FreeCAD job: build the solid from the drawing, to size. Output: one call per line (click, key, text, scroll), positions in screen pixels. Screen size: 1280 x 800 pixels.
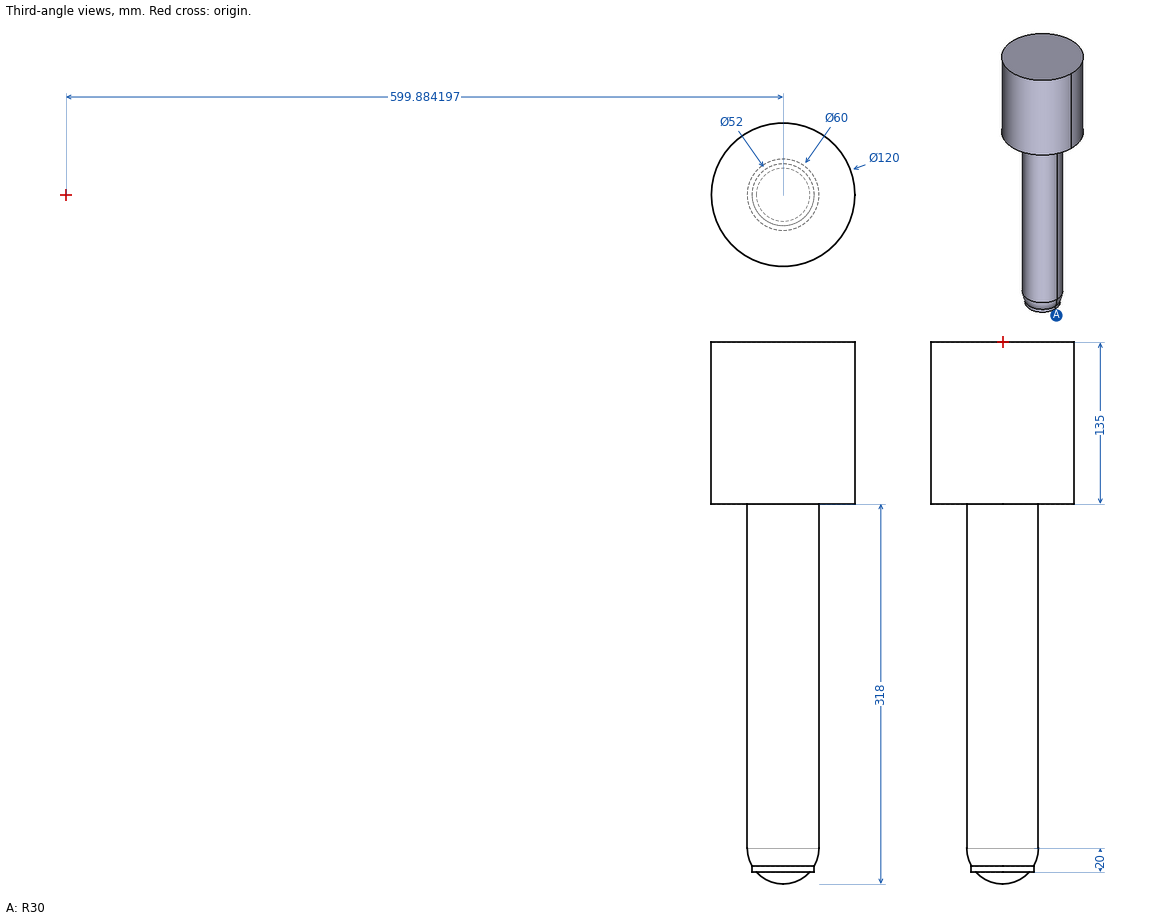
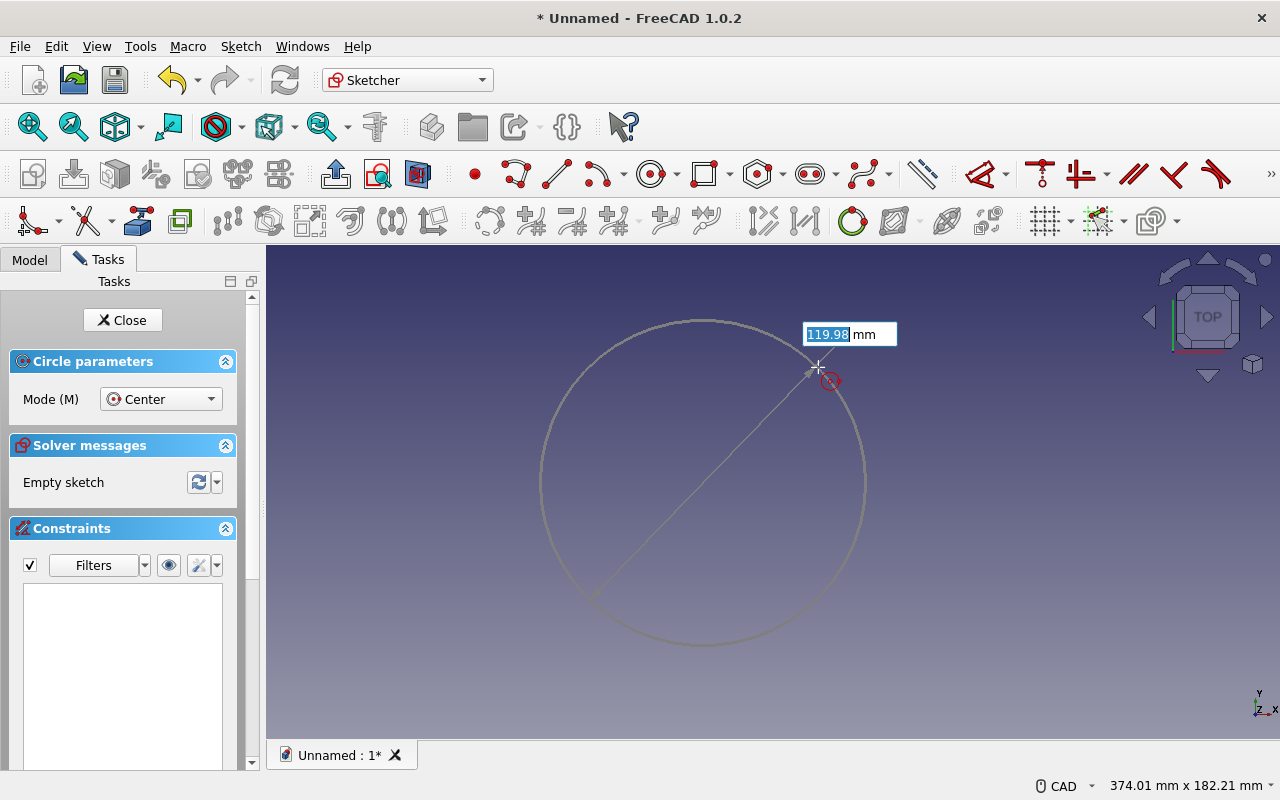
text(120)
key(Return)
key(Escape)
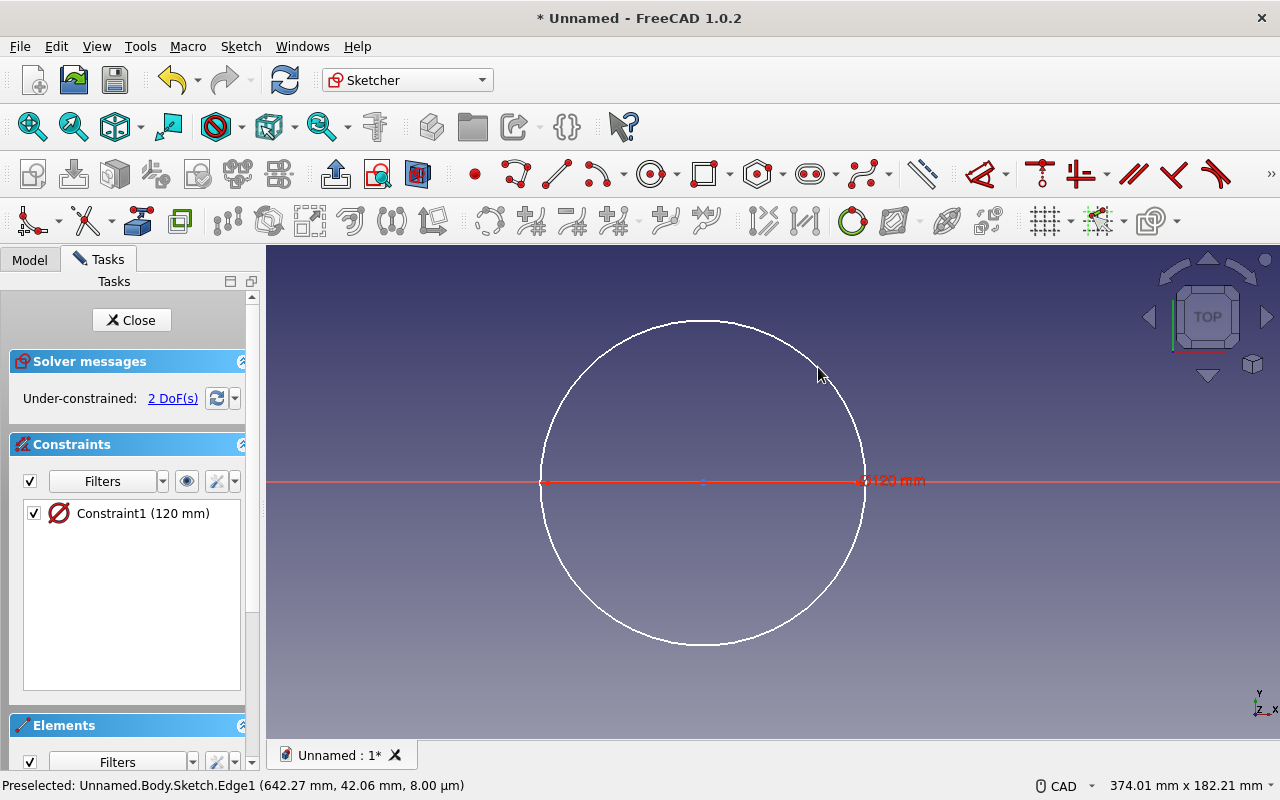
click(703, 483)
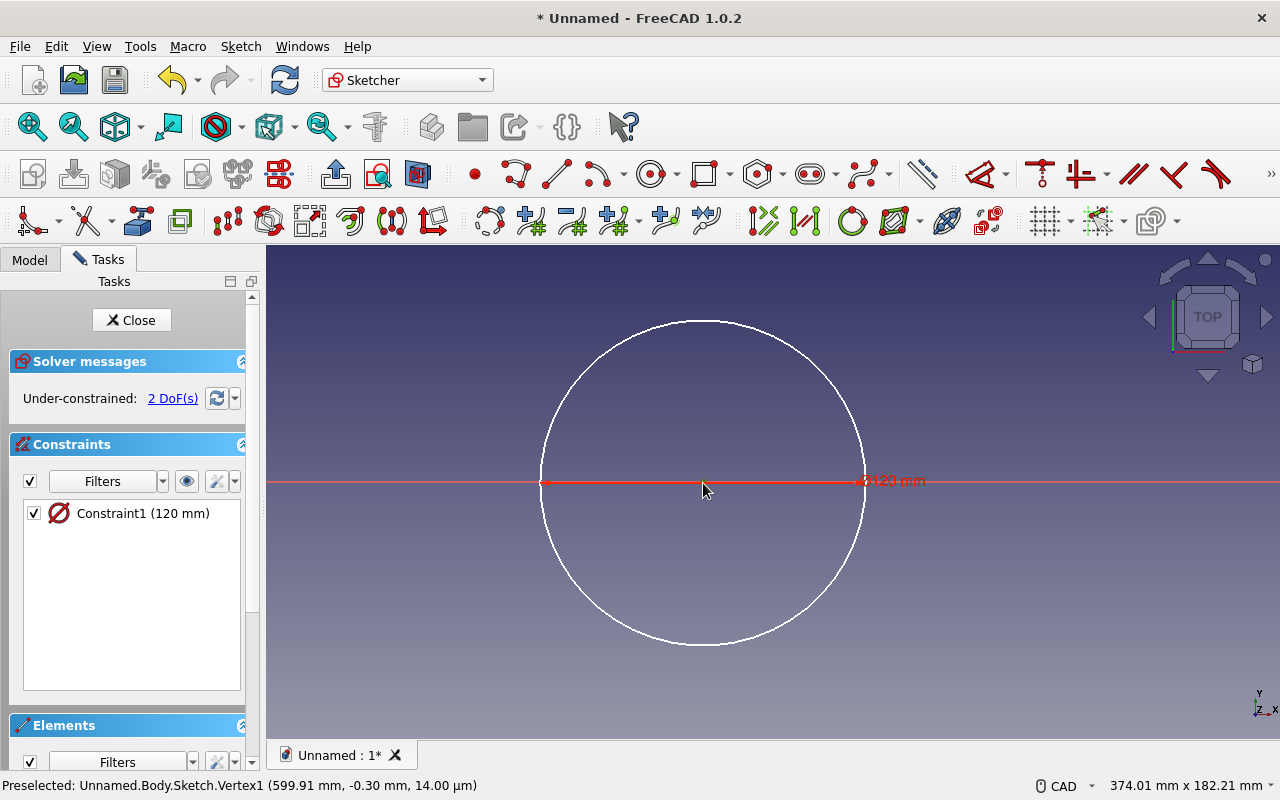
click(353, 482)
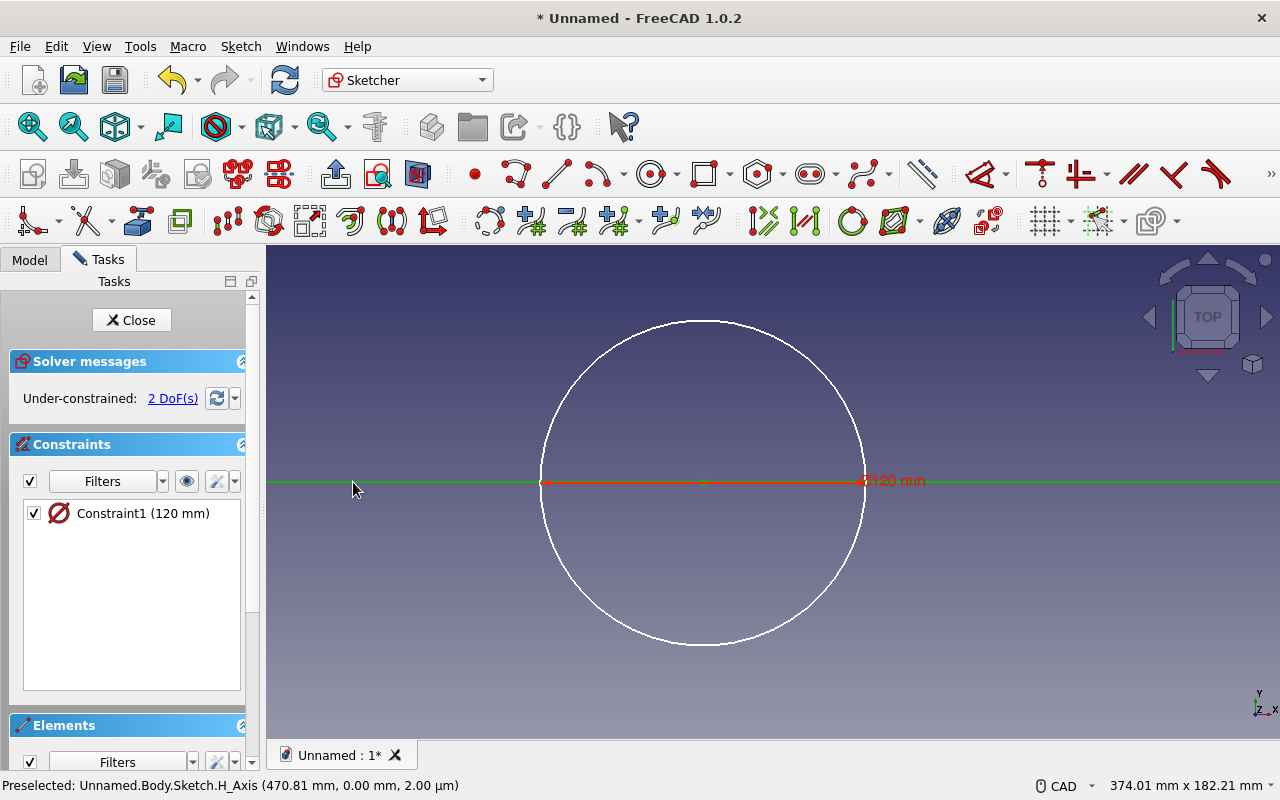
click(1040, 174)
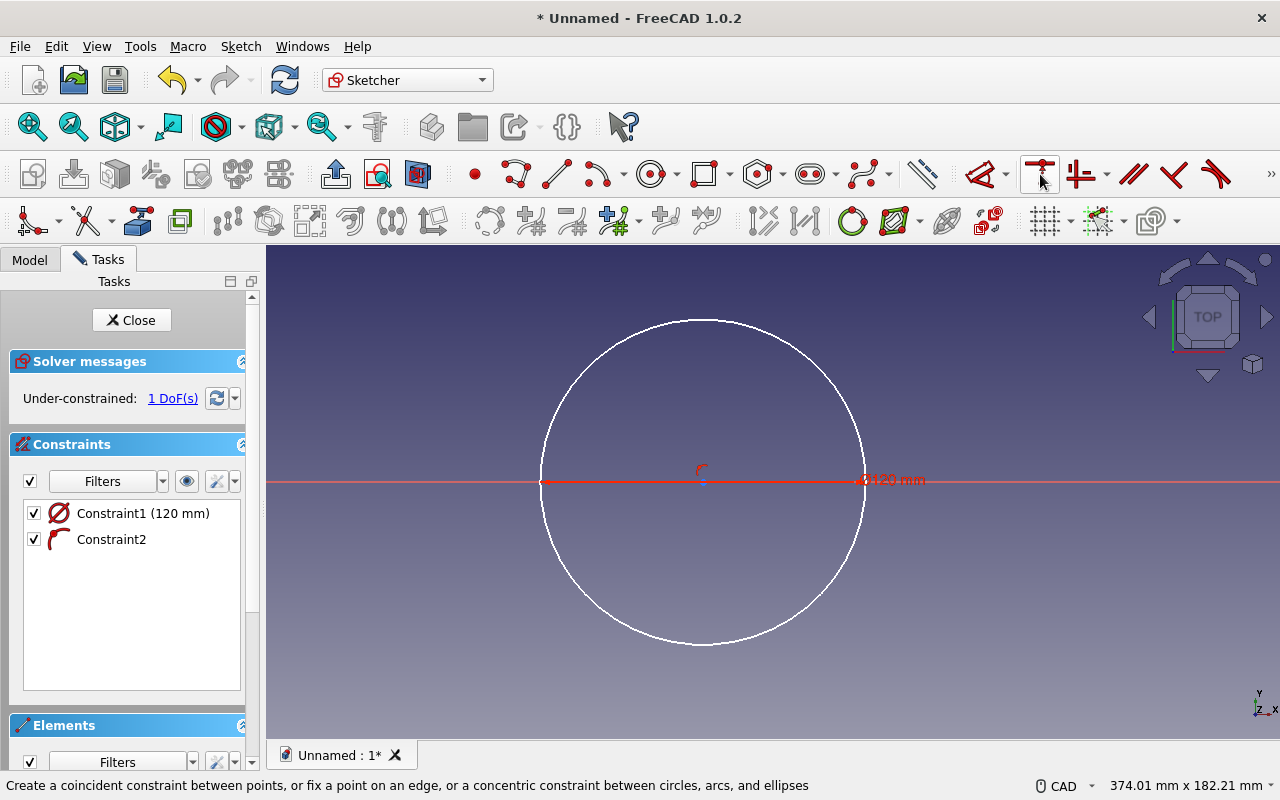
click(980, 174)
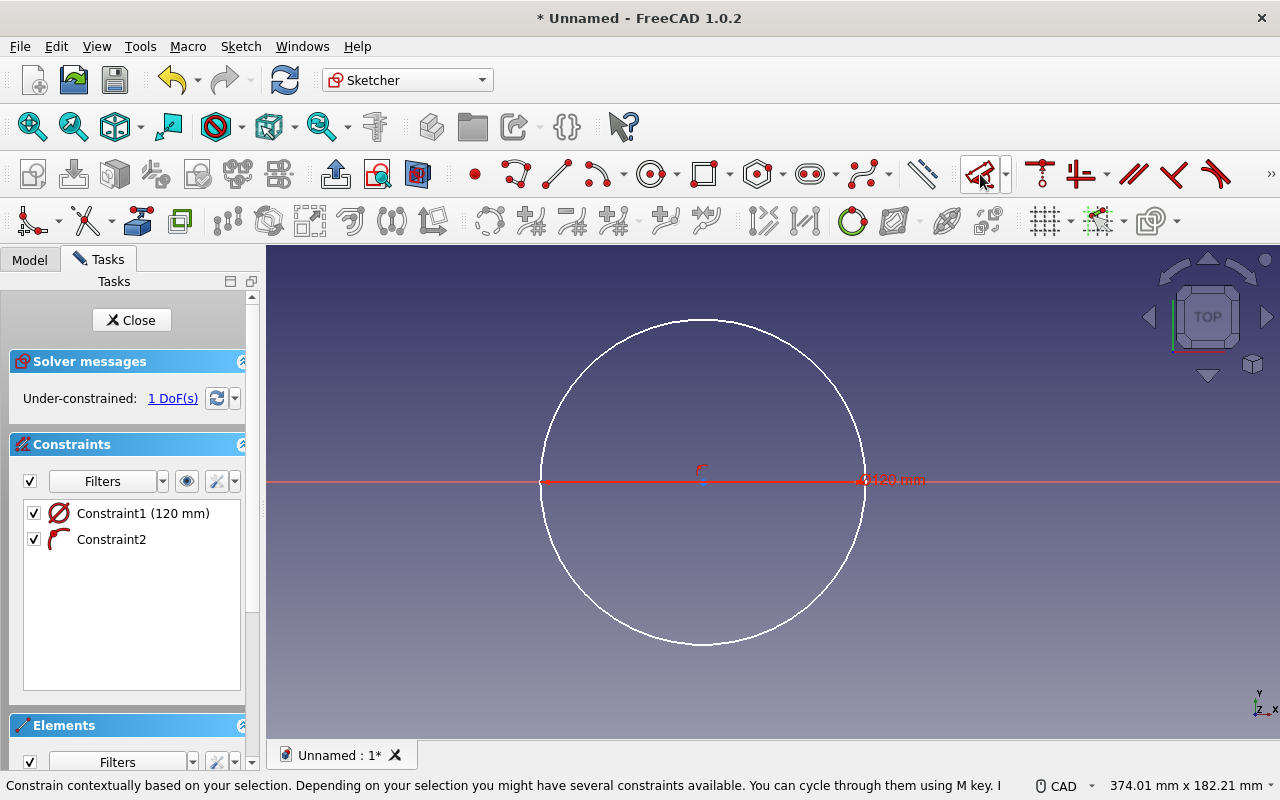
click(703, 482)
click(498, 516)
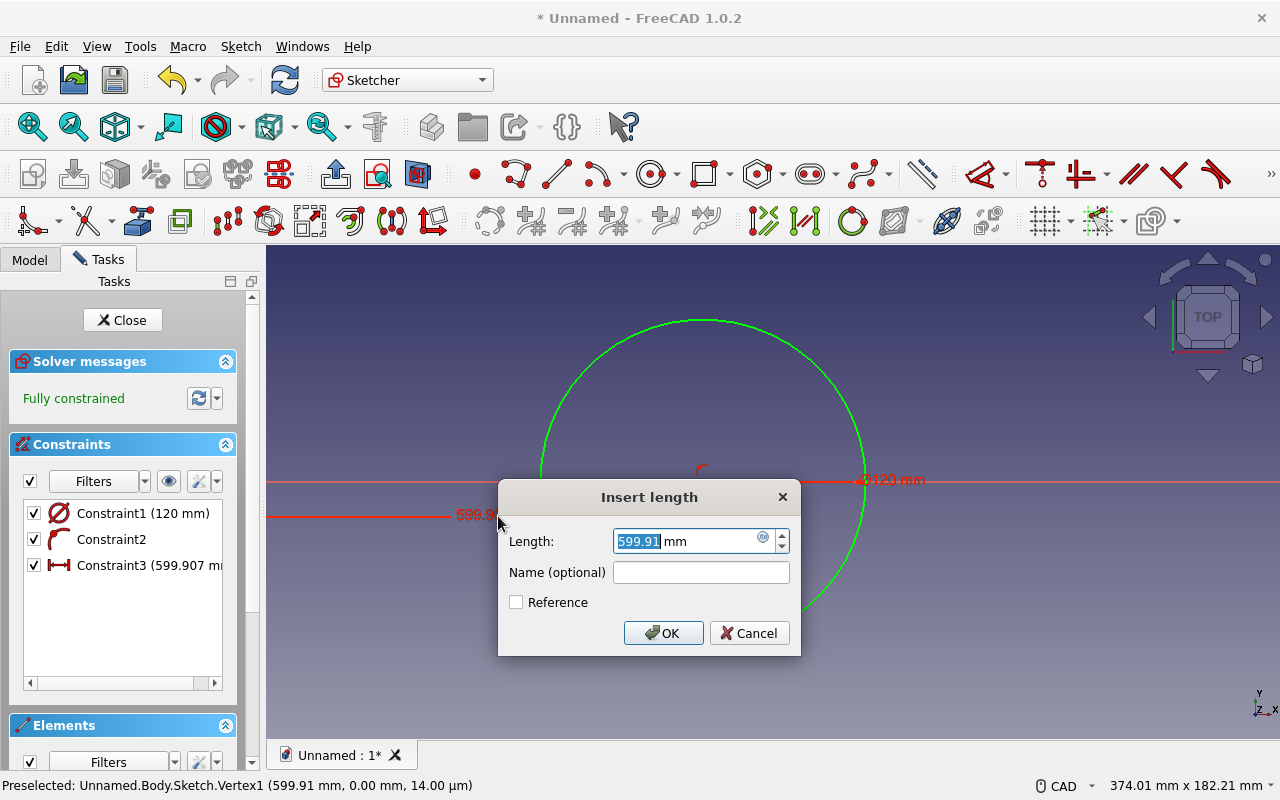
text(599.884197)
key(Return)
key(Escape)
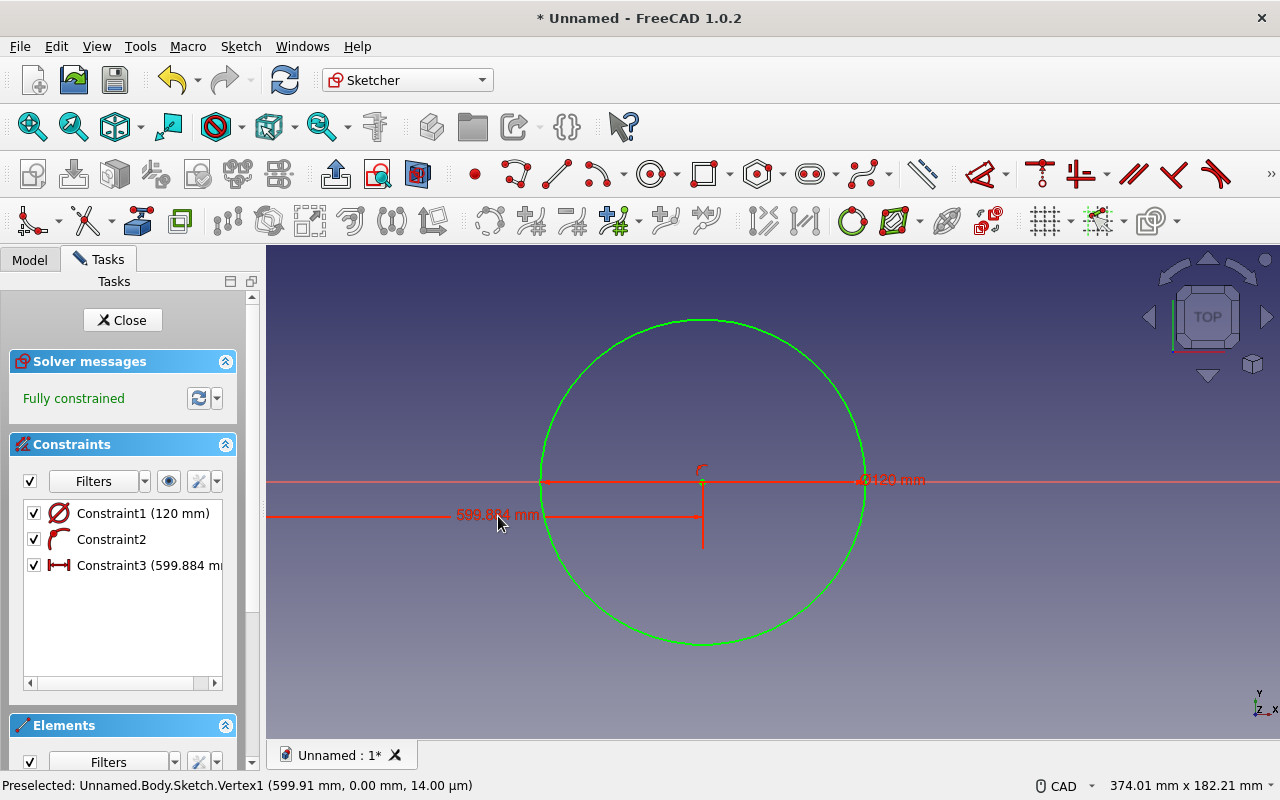
click(123, 320)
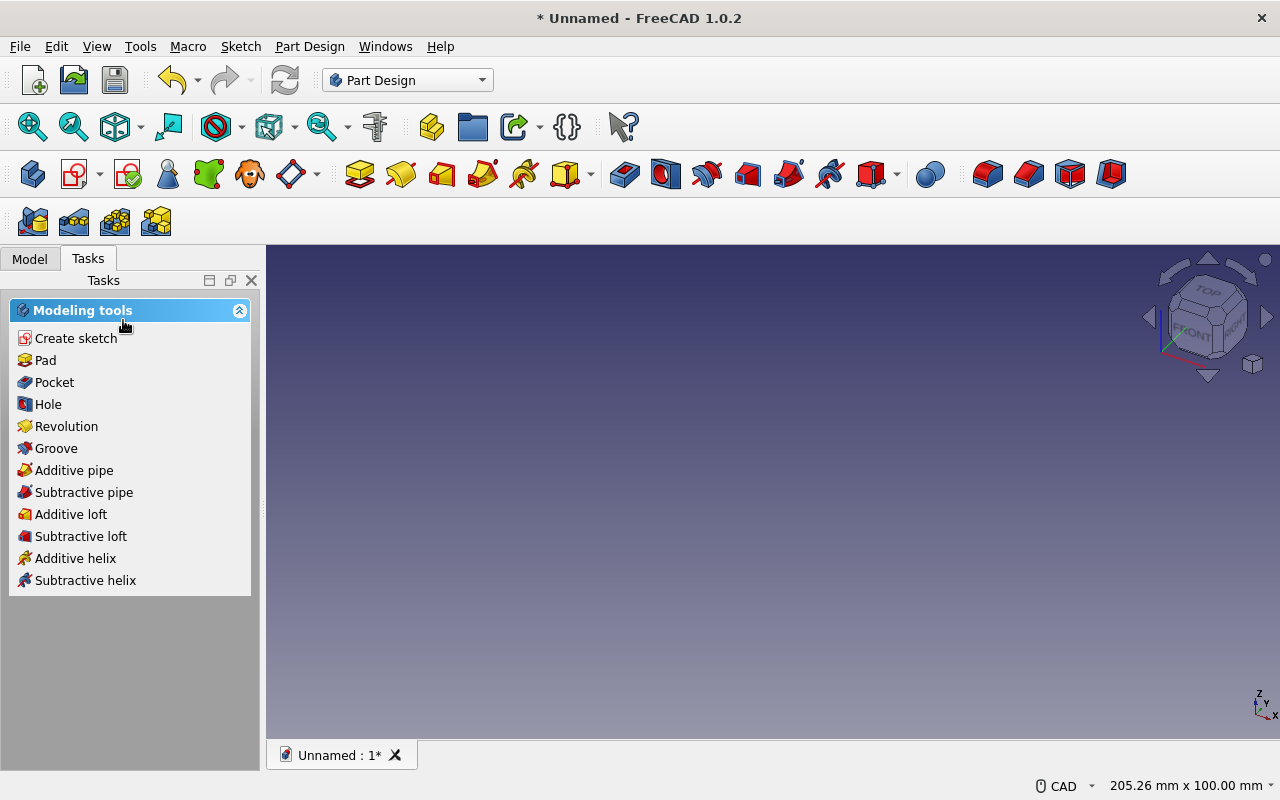
click(360, 174)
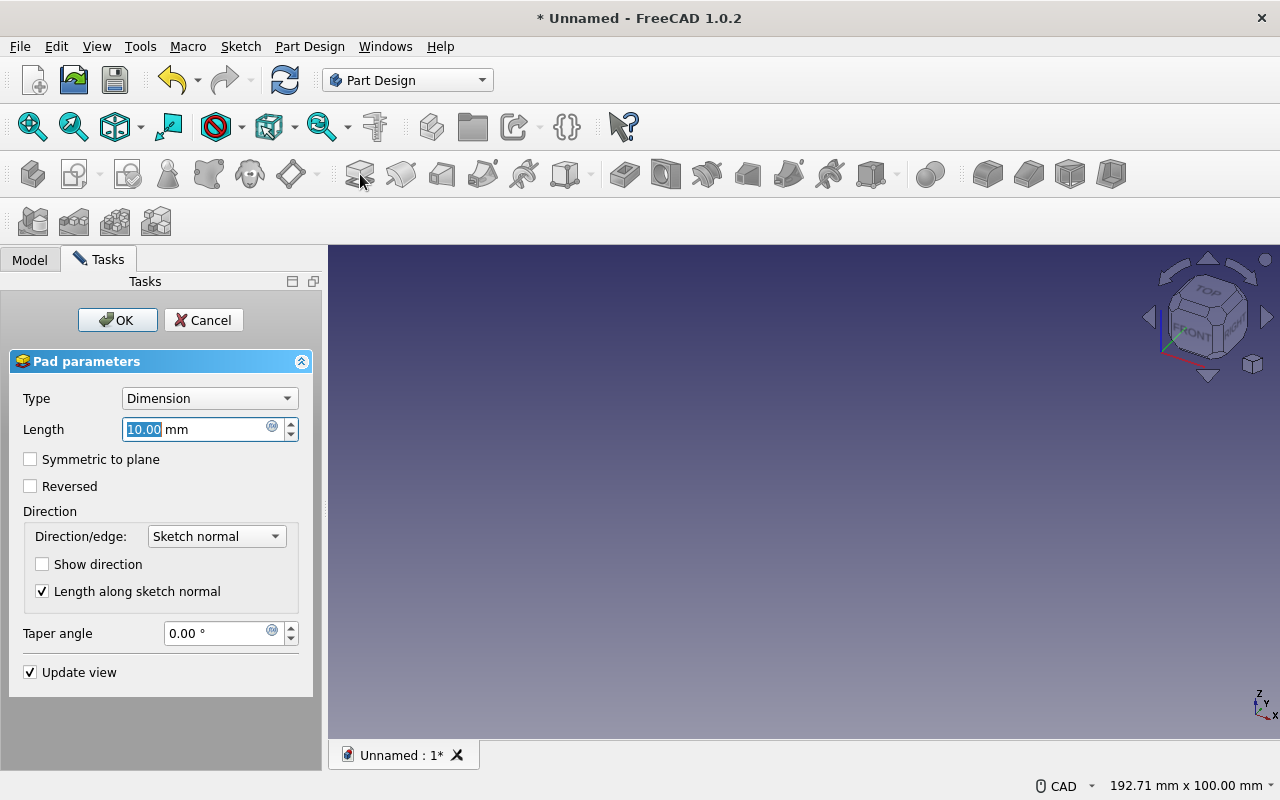
text(135)
key(Tab)